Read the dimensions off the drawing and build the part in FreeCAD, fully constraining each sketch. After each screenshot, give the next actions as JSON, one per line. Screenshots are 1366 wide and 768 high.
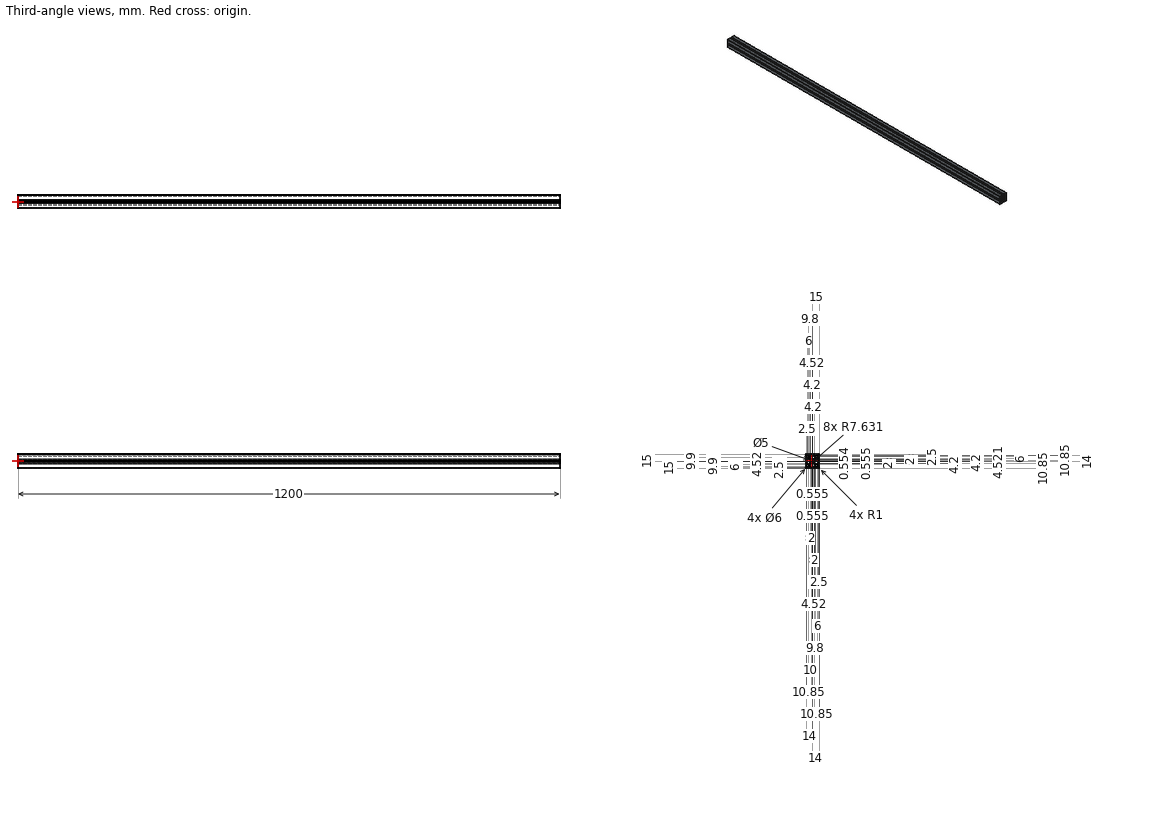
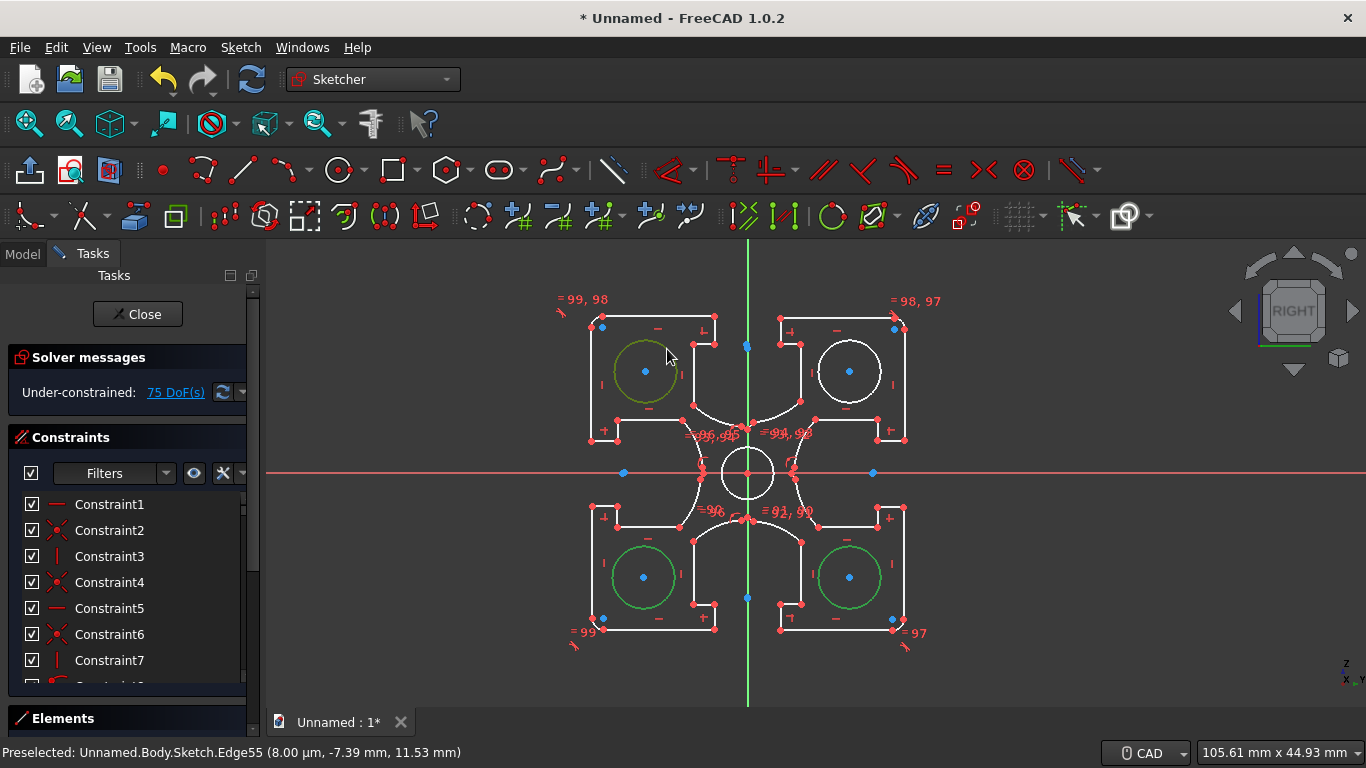
{"action": "left_click", "coordinate": [871, 349]}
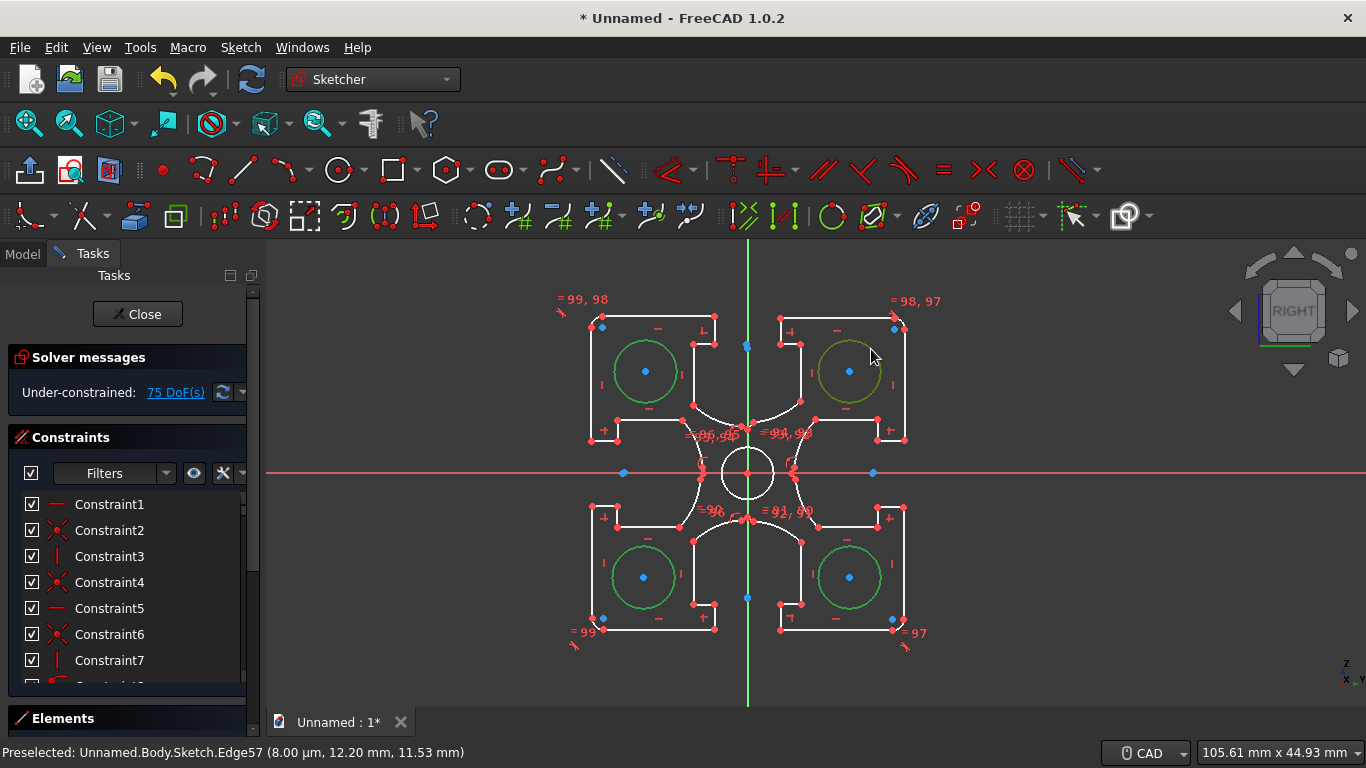
{"action": "left_click", "coordinate": [944, 170]}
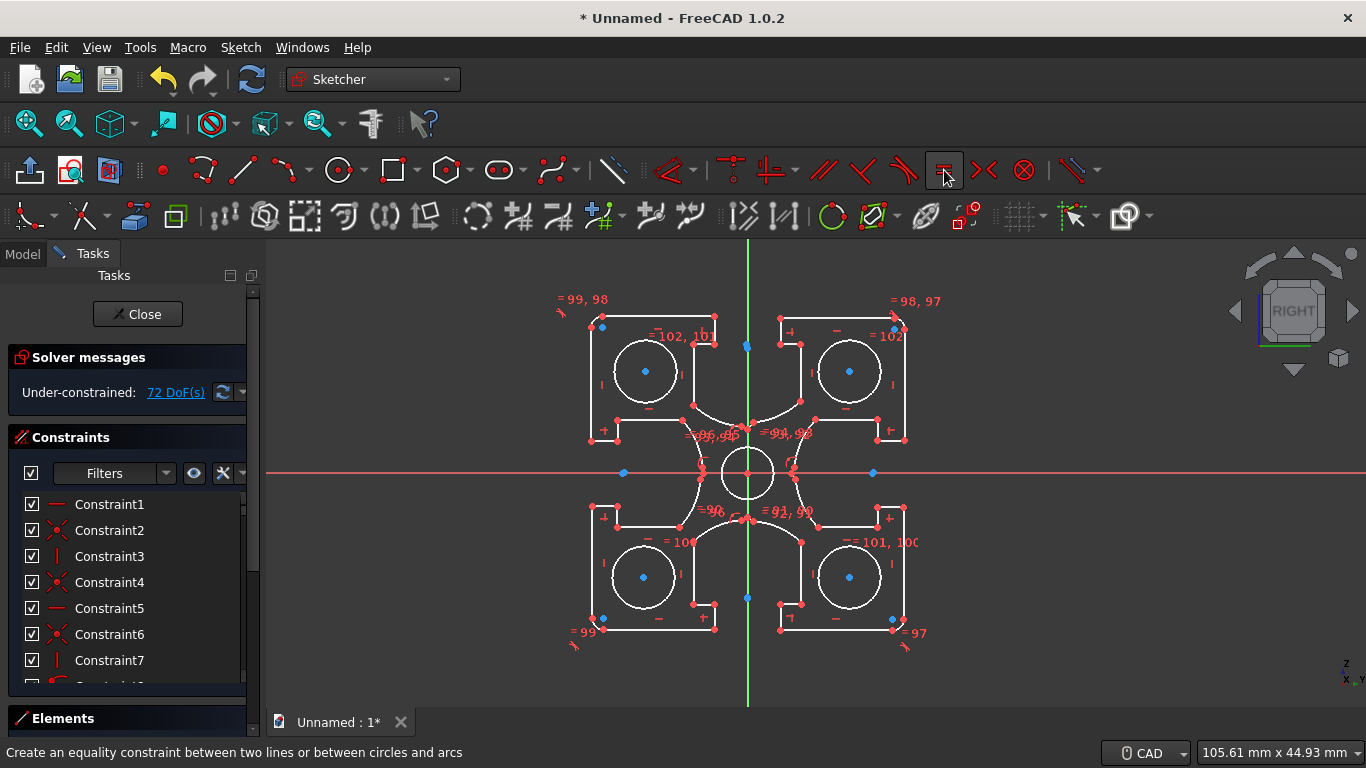
{"action": "left_click", "coordinate": [668, 170]}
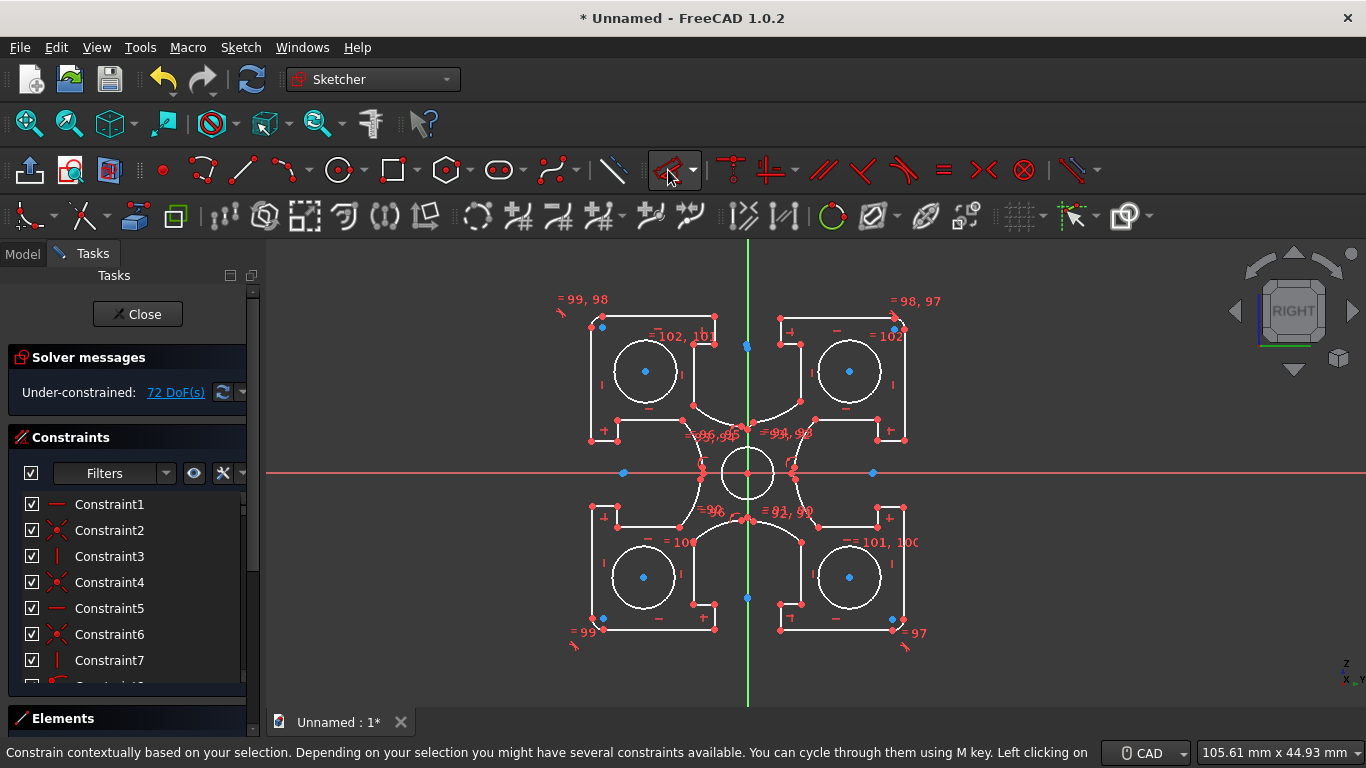
{"action": "left_click", "coordinate": [726, 523]}
{"action": "left_click", "coordinate": [642, 566]}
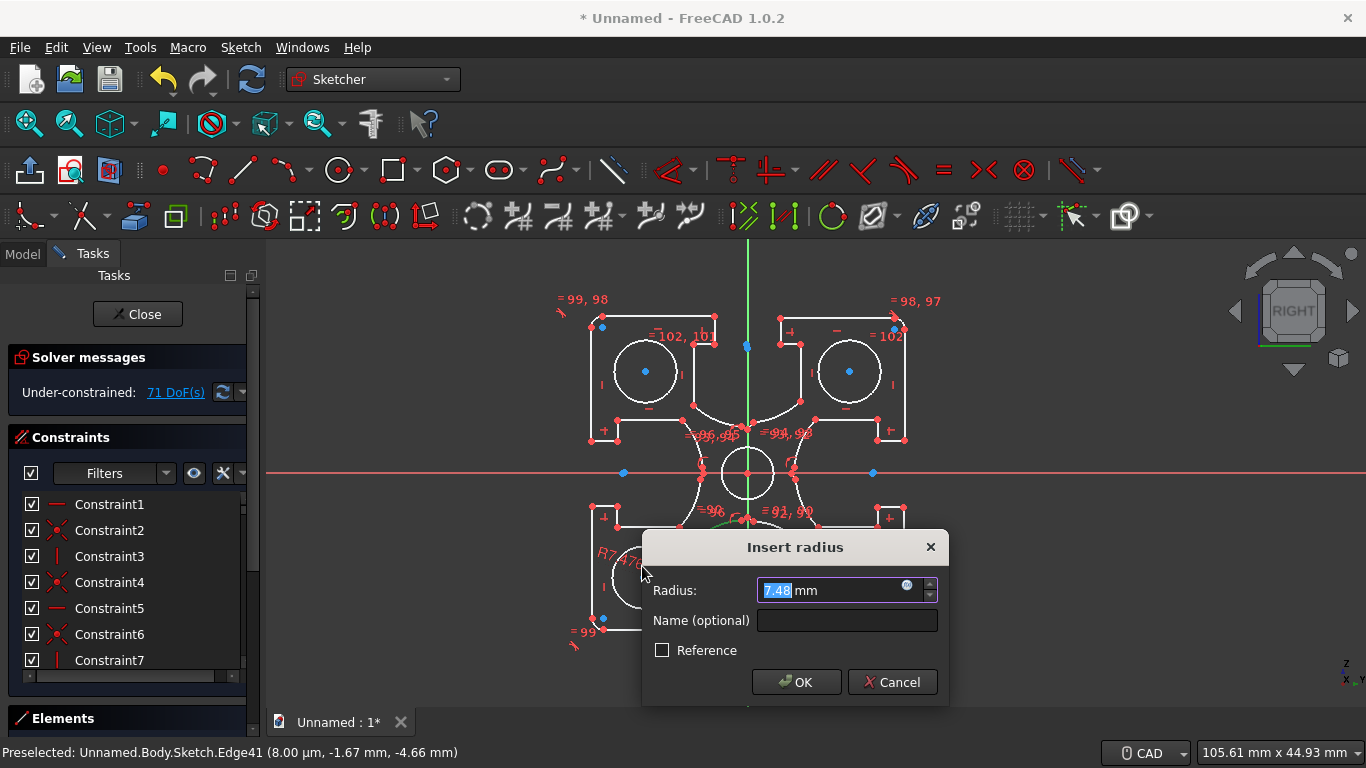
{"action": "type", "text": "7.631"}
{"action": "key", "text": "Return"}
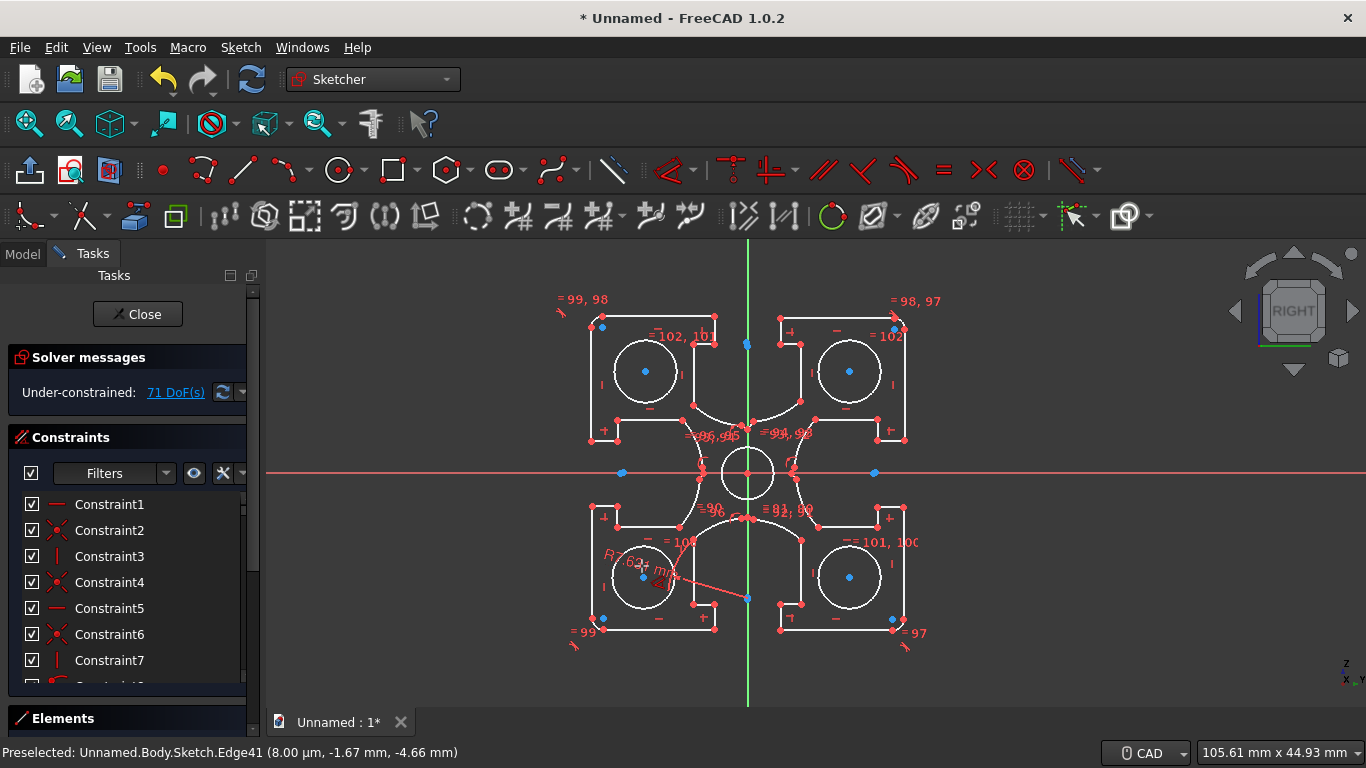
{"action": "scroll", "coordinate": [901, 627], "scroll_direction": "up", "scroll_amount": 7}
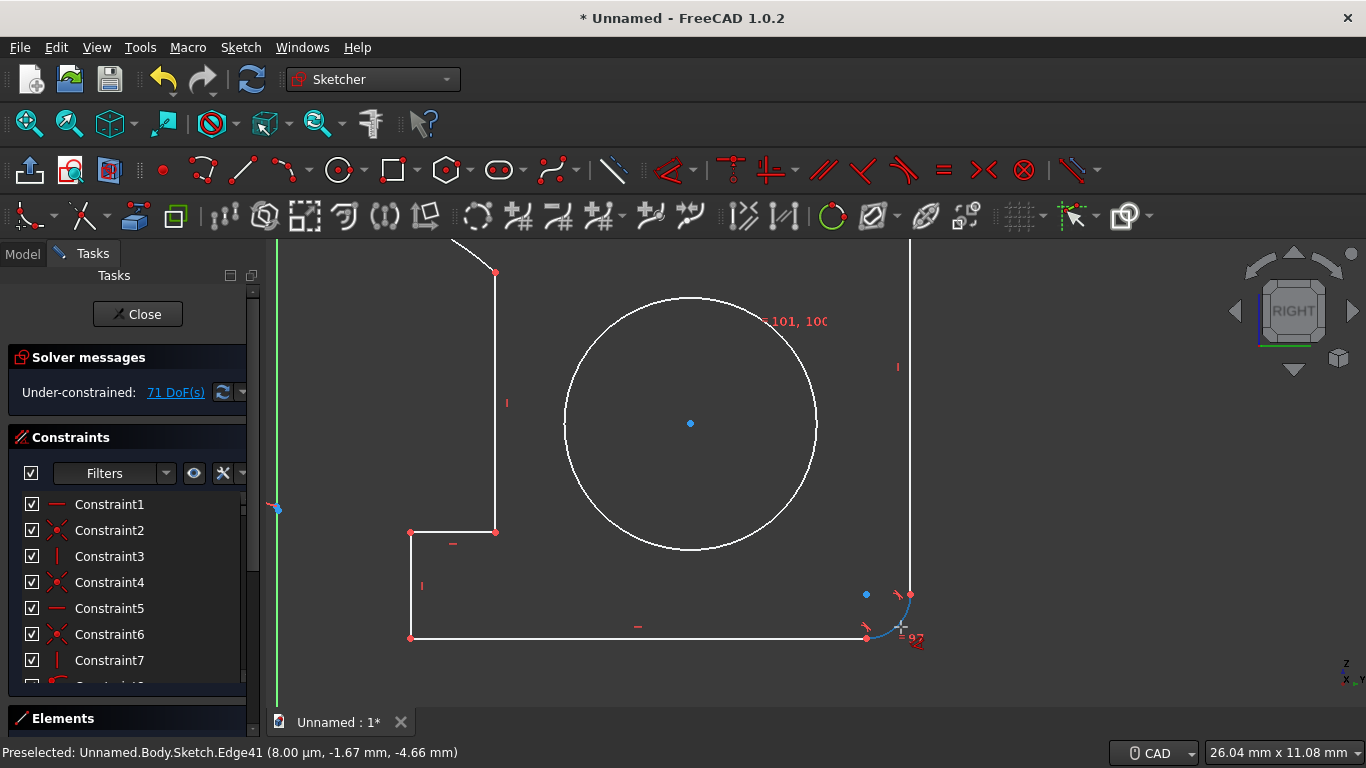
{"action": "left_click", "coordinate": [898, 626]}
{"action": "left_click", "coordinate": [921, 649]}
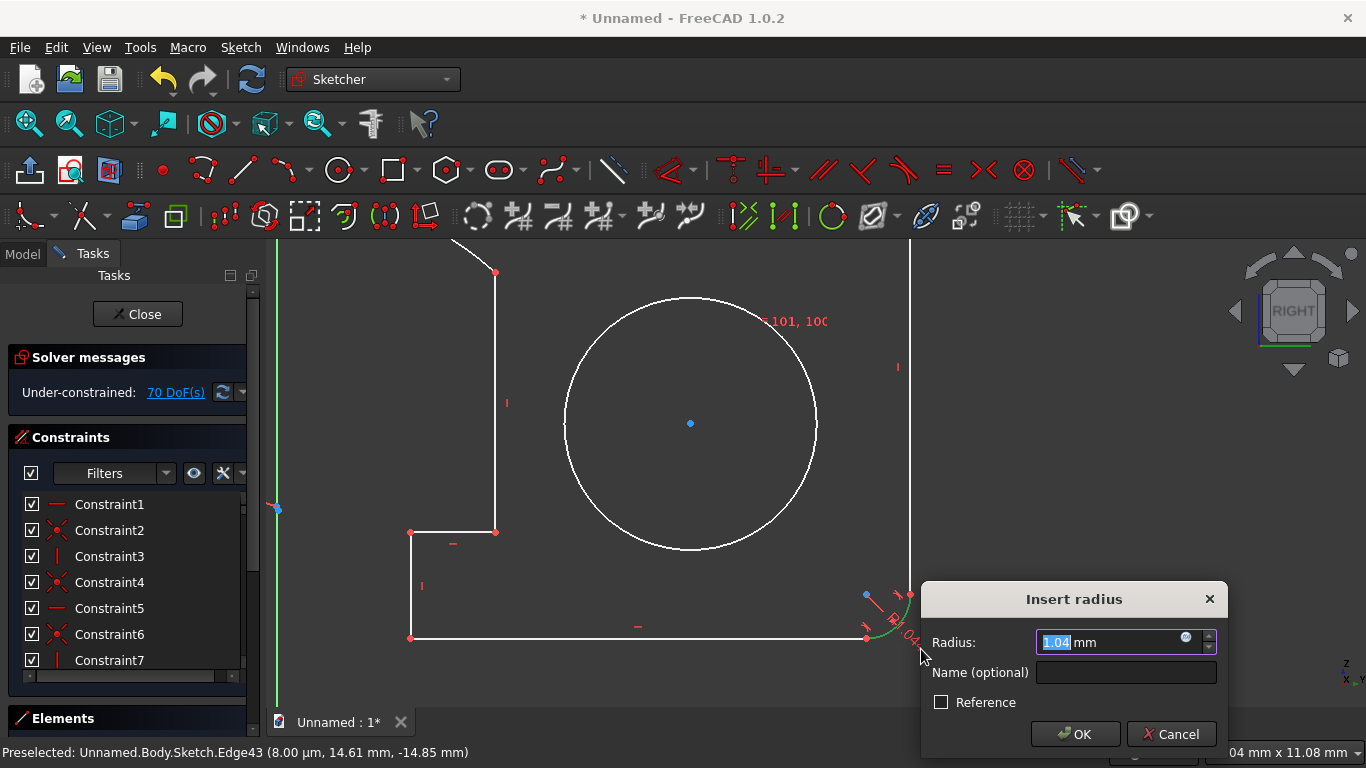
{"action": "type", "text": "1"}
{"action": "key", "text": "Return"}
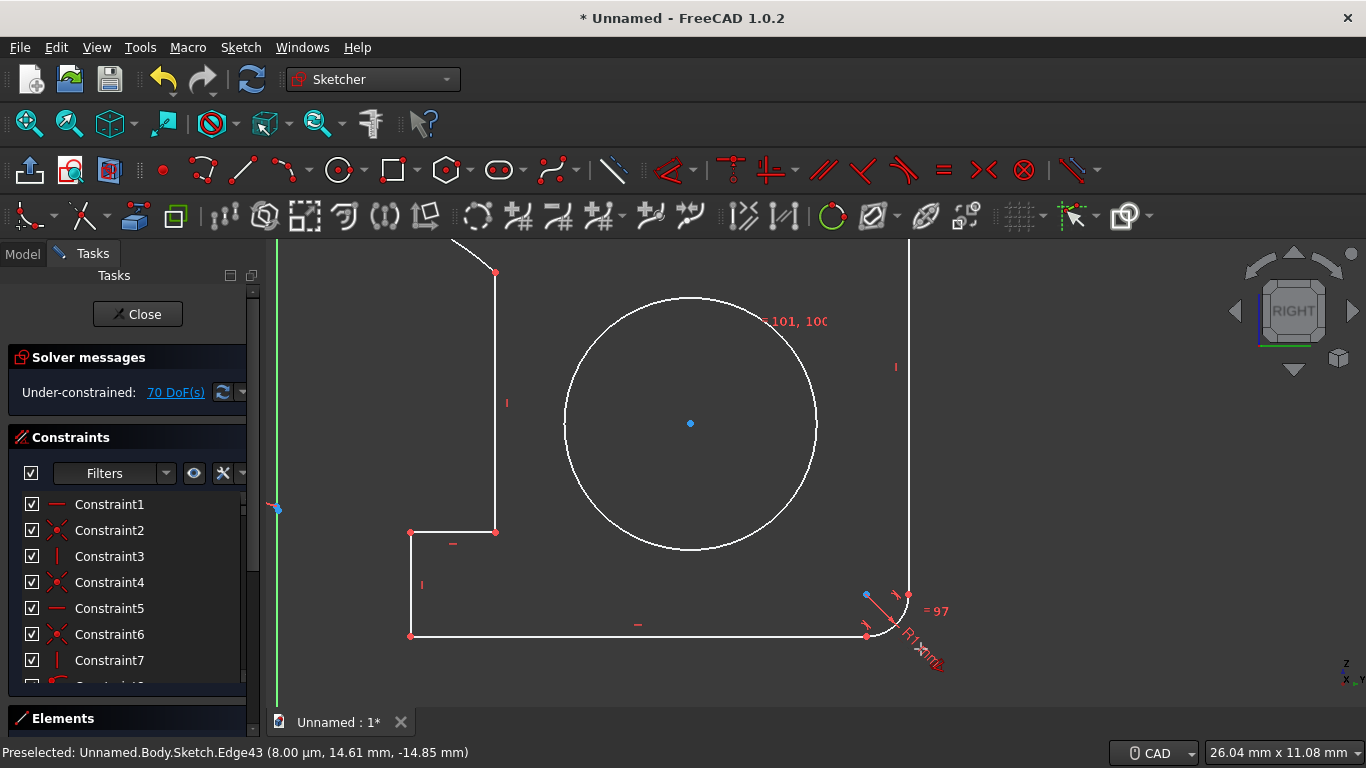
{"action": "scroll", "coordinate": [901, 627], "scroll_direction": "down", "scroll_amount": 7}